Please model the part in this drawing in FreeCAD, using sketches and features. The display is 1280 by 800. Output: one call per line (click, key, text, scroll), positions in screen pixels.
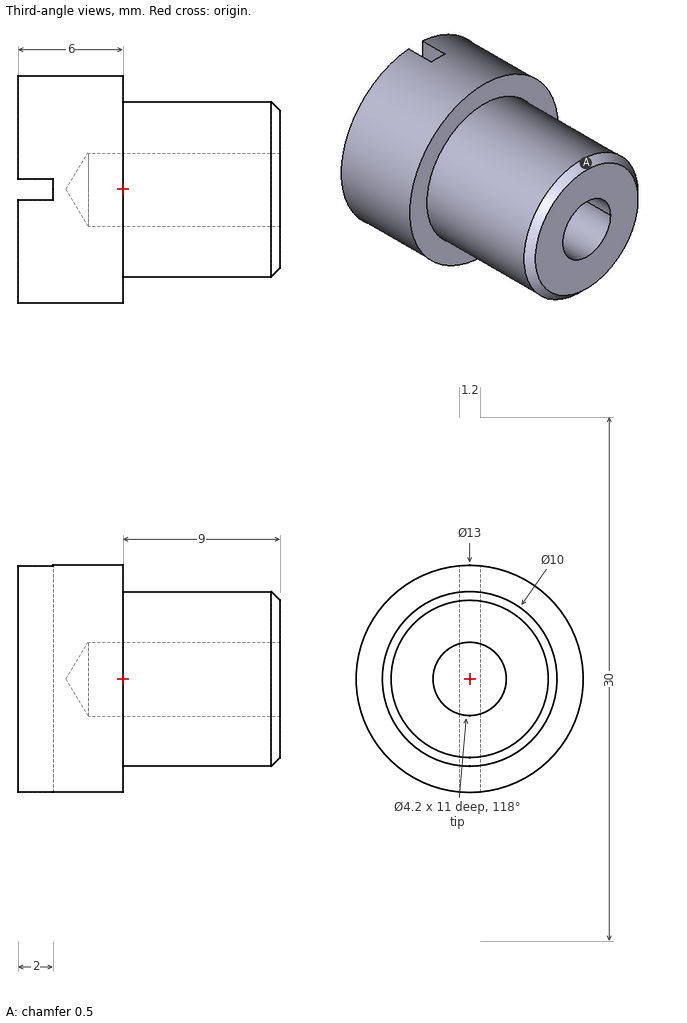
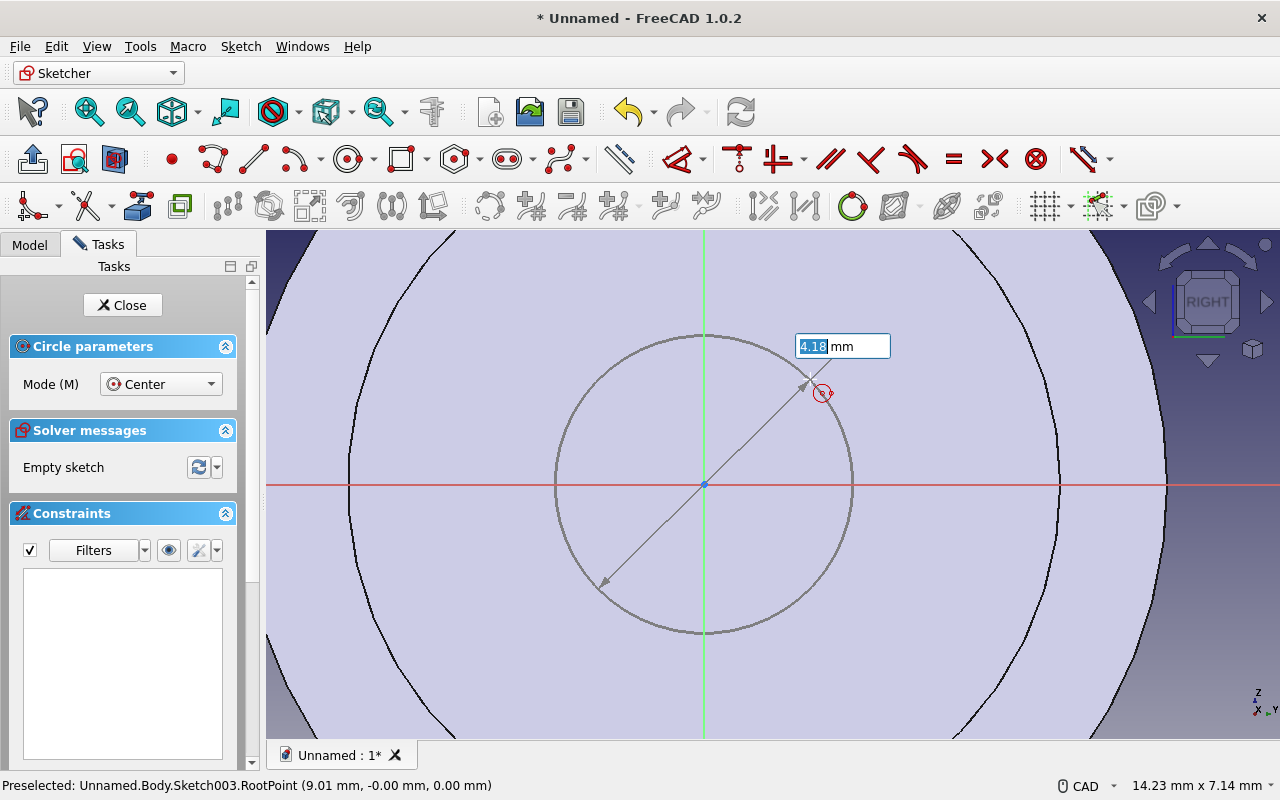
text(4.2)
key(Return)
key(Escape)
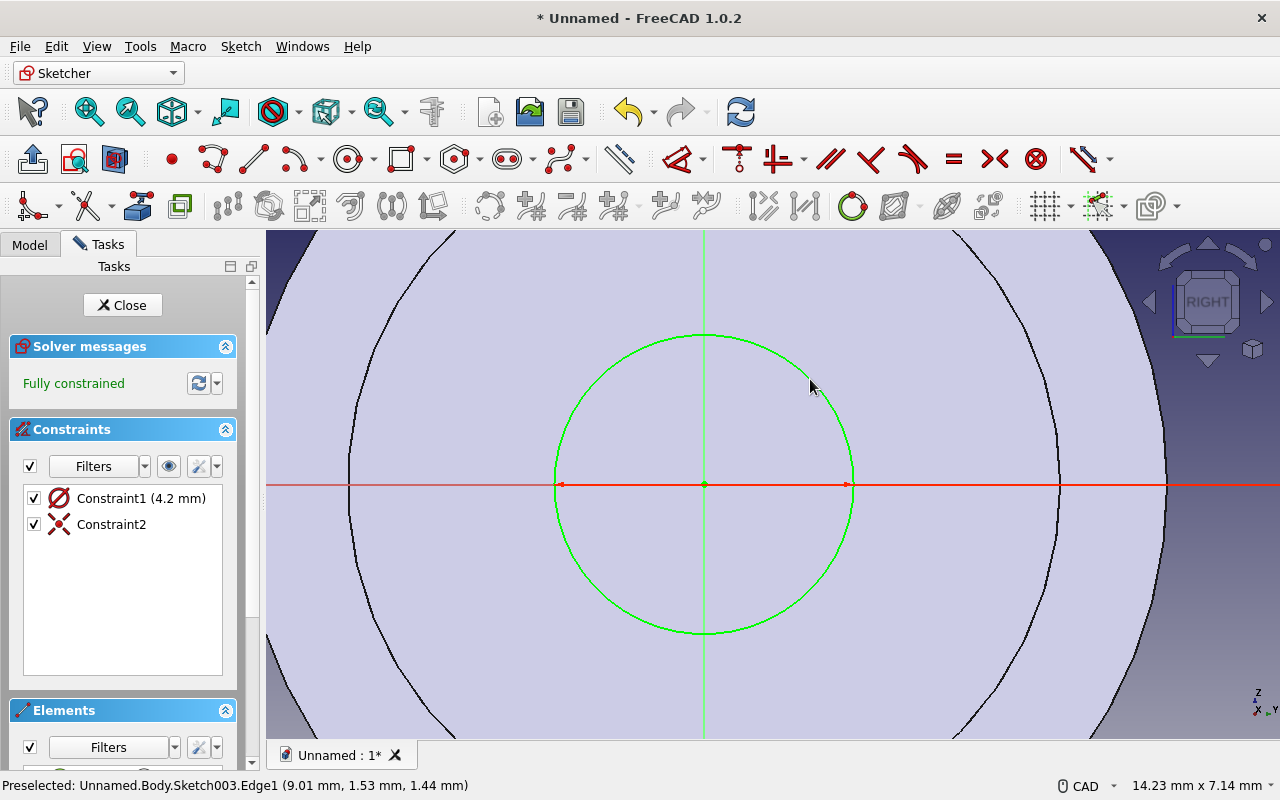
click(123, 305)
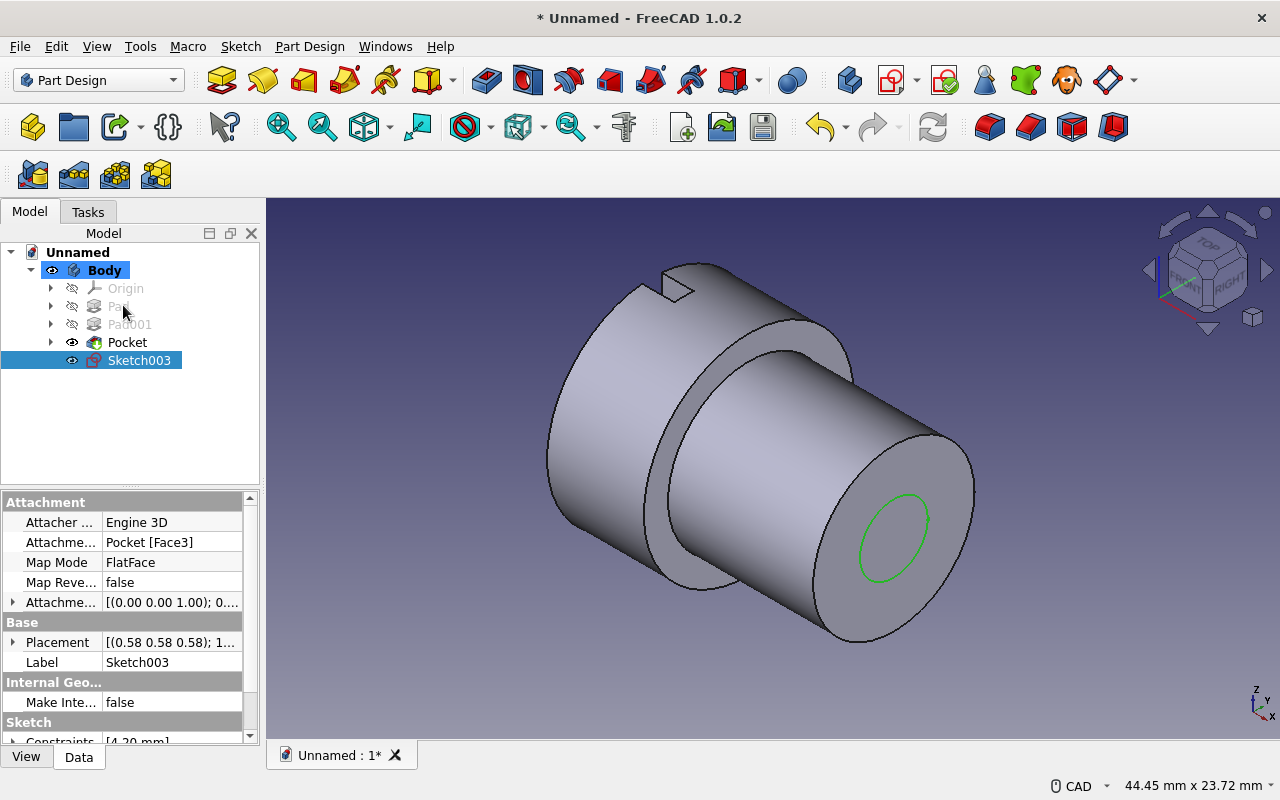
click(528, 80)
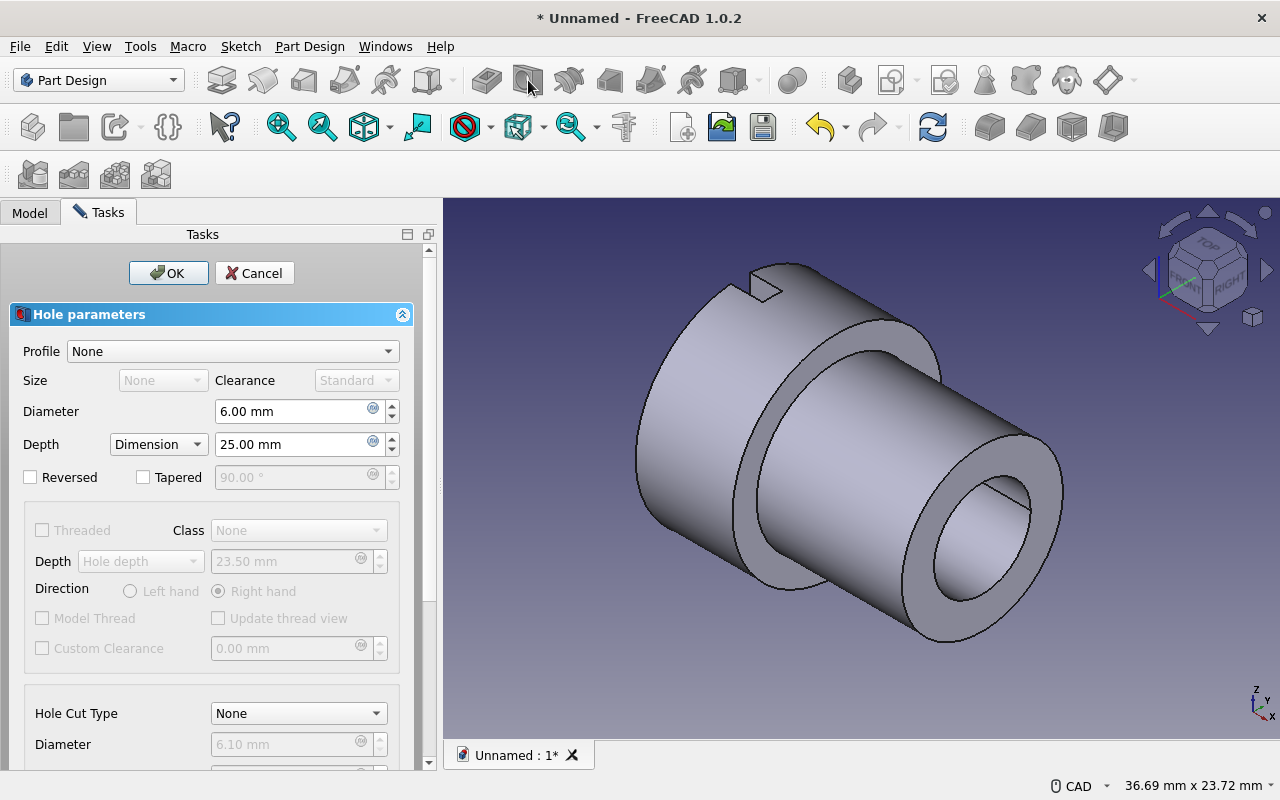
triple_click(300, 412)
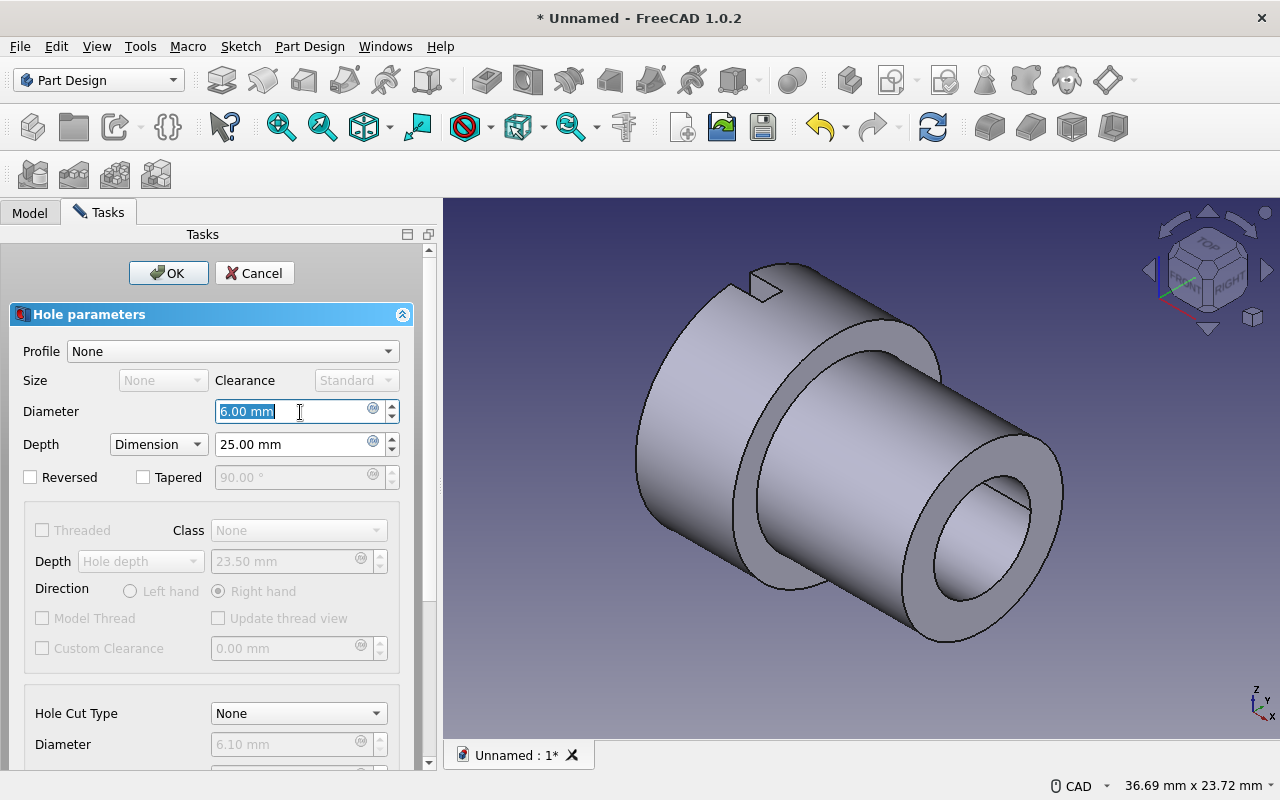
text(4.2)
key(Tab)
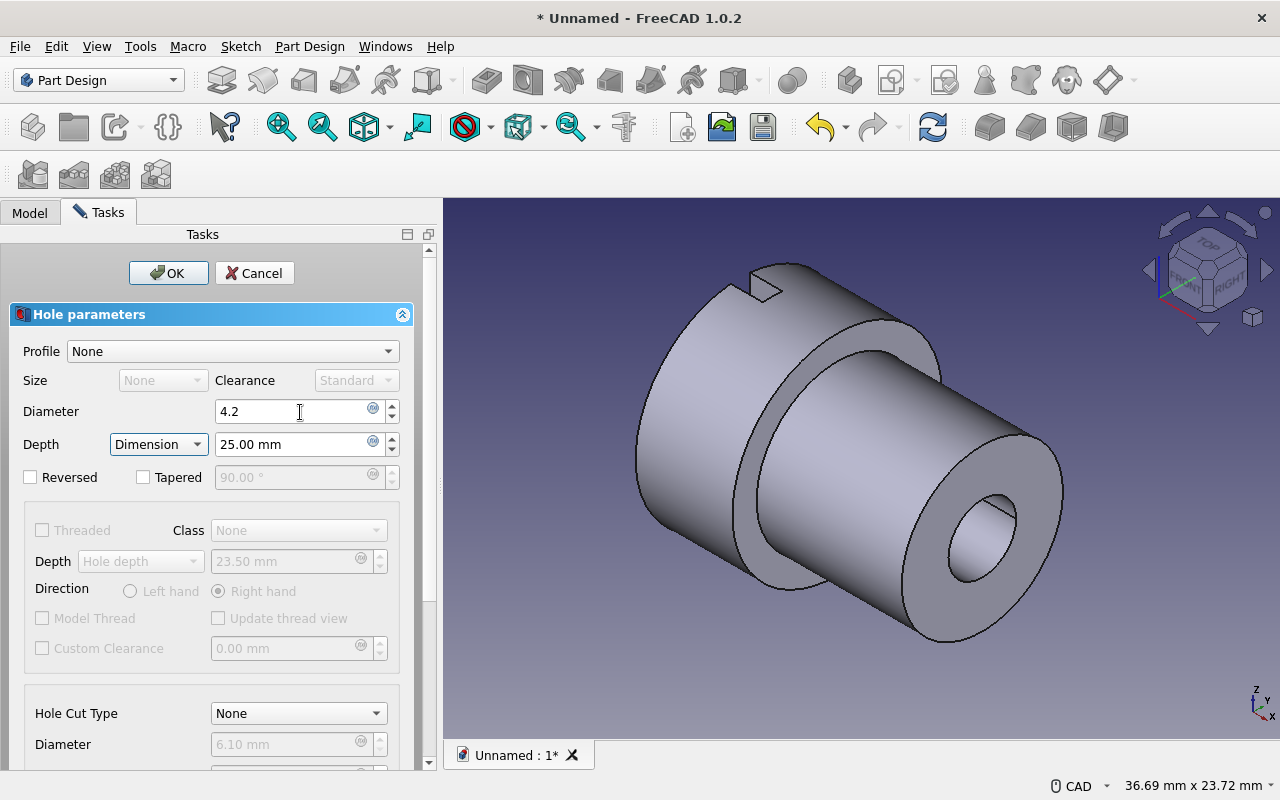
triple_click(300, 444)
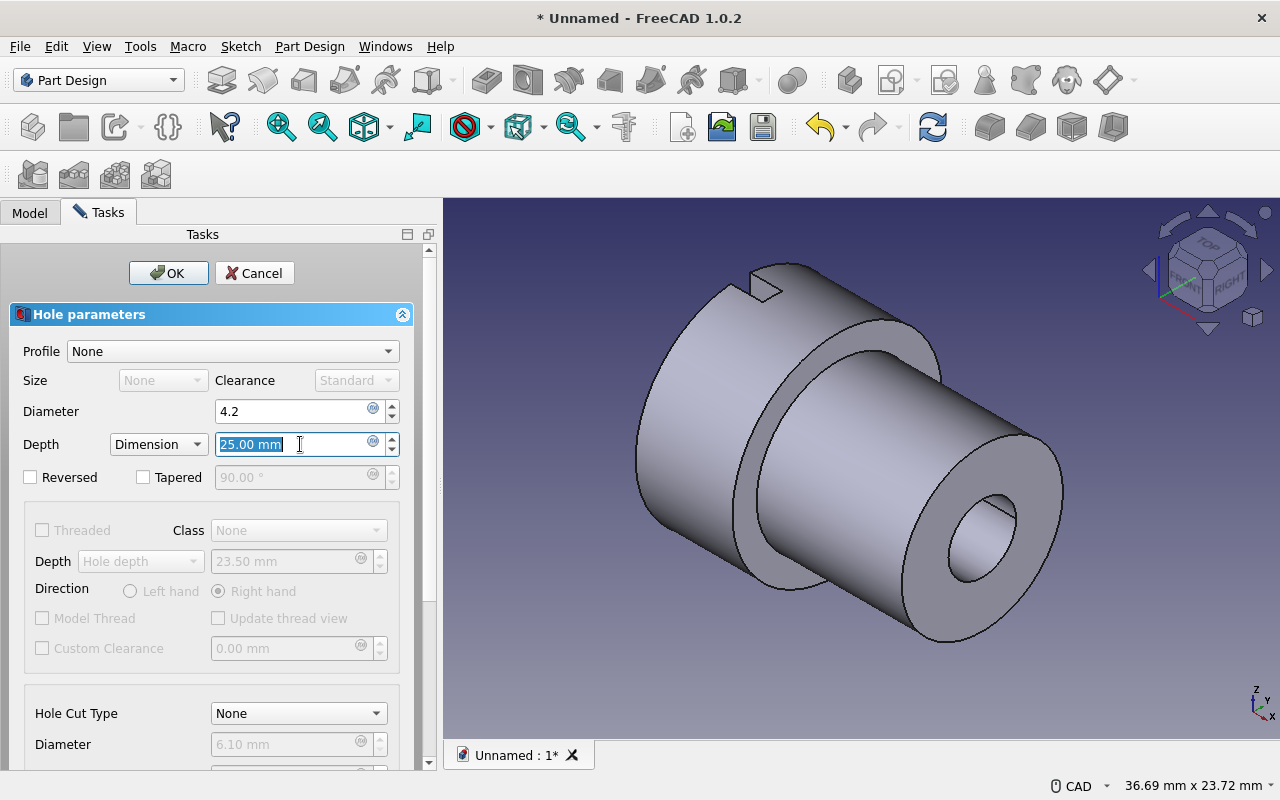
text(11)
key(Tab)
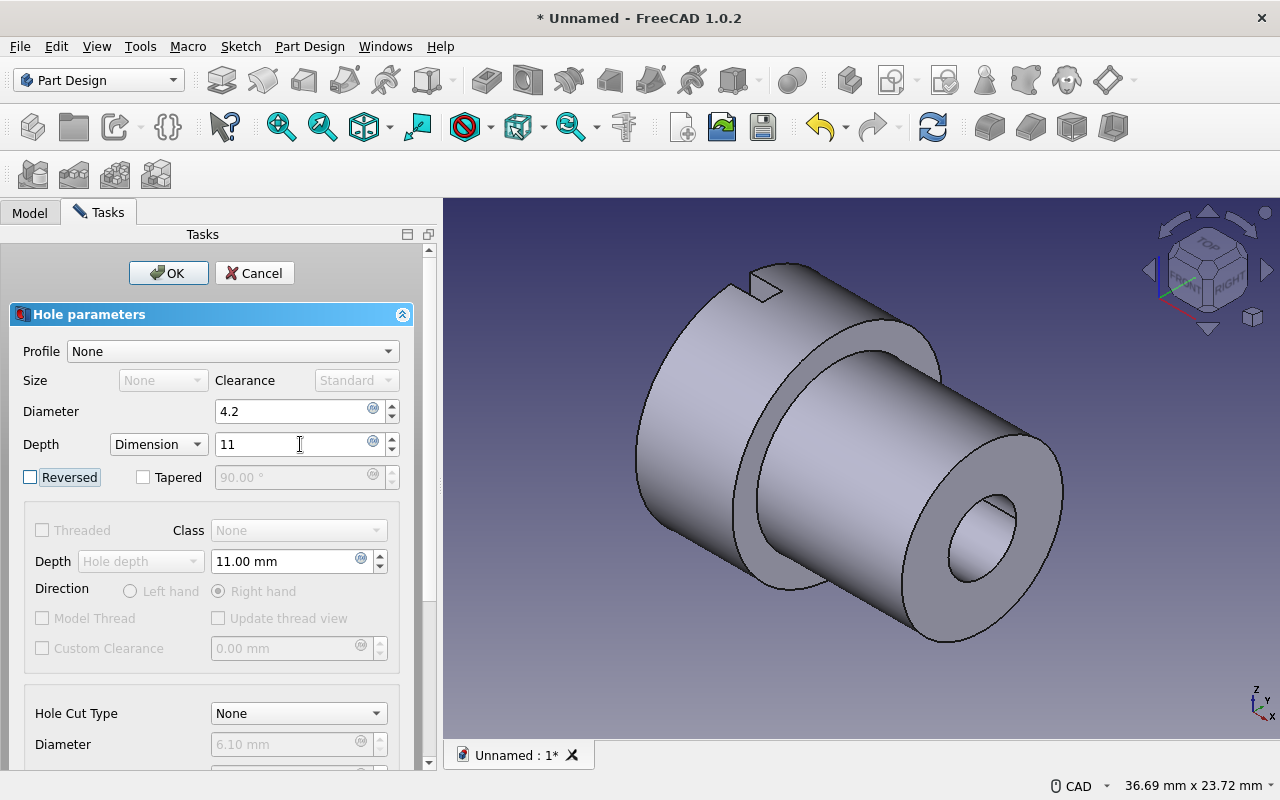
click(169, 273)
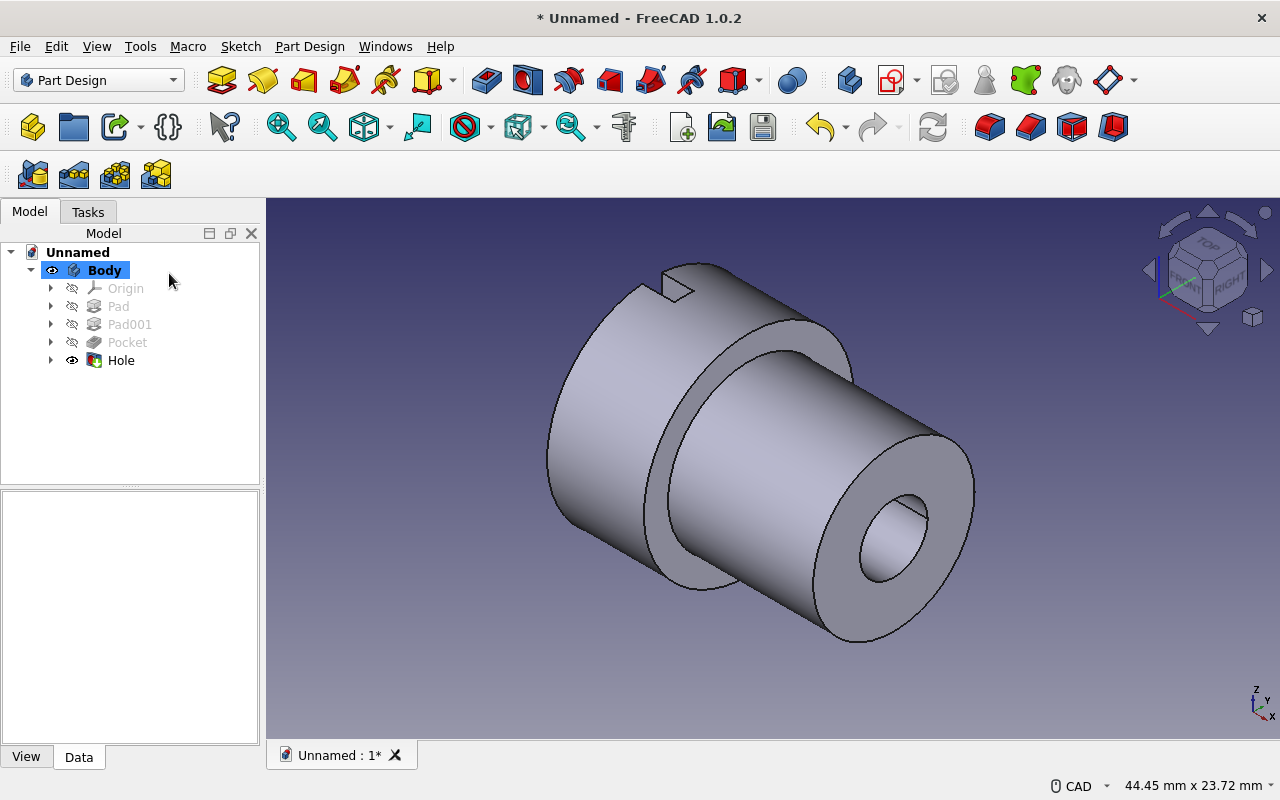
click(813, 584)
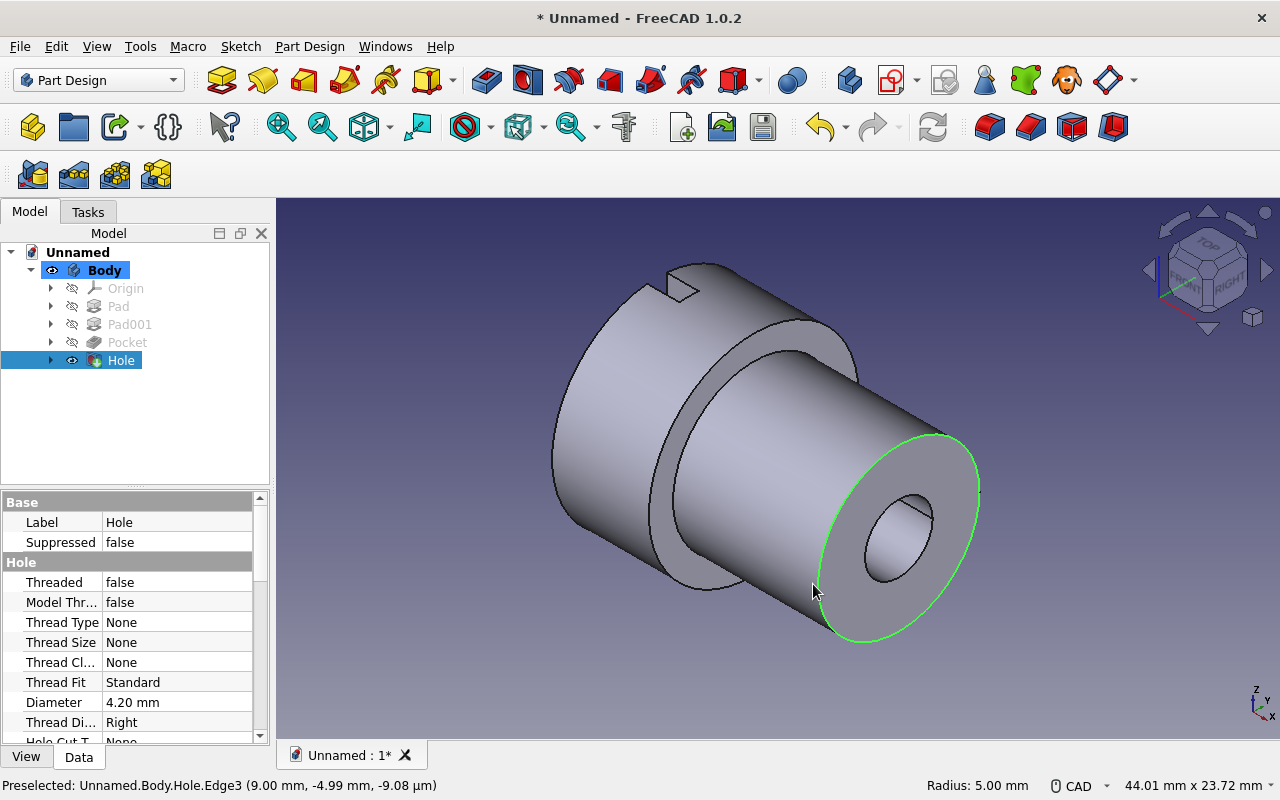
click(1031, 128)